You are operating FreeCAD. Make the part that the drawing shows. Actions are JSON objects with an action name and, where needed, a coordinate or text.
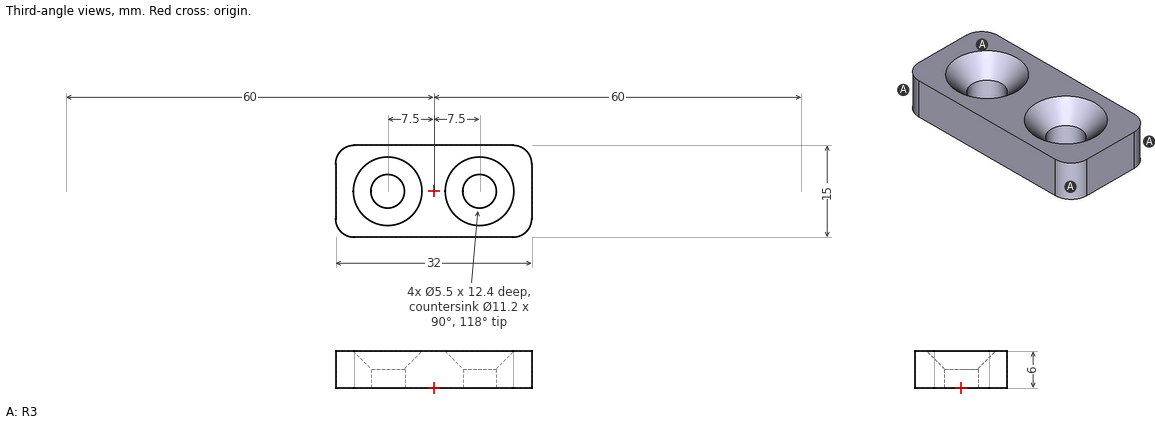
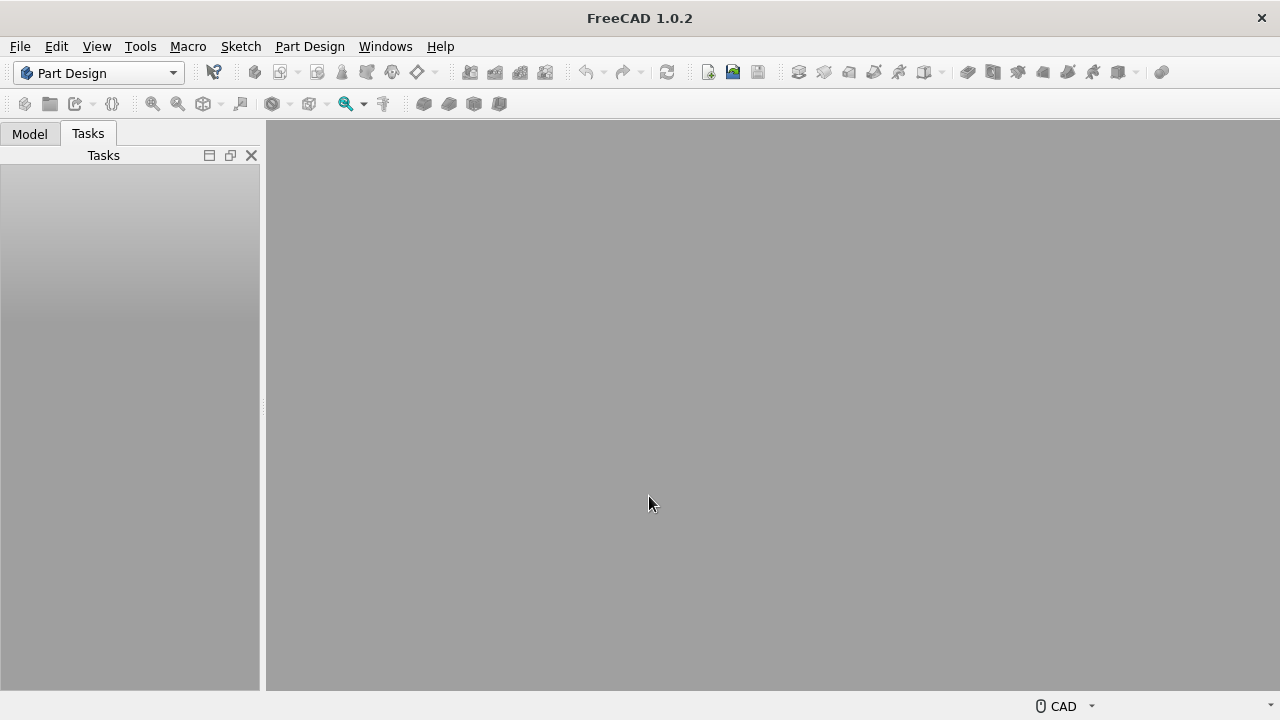
{"action": "left_click", "coordinate": [708, 72]}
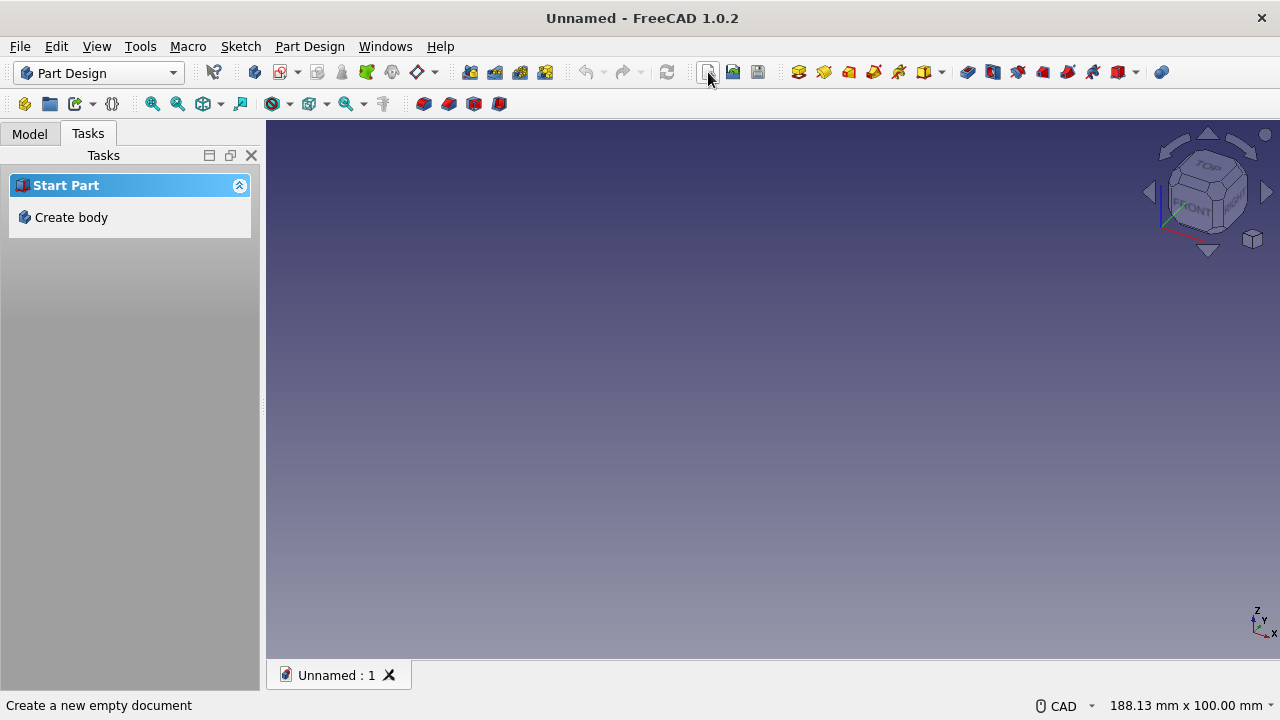
{"action": "left_click", "coordinate": [280, 72]}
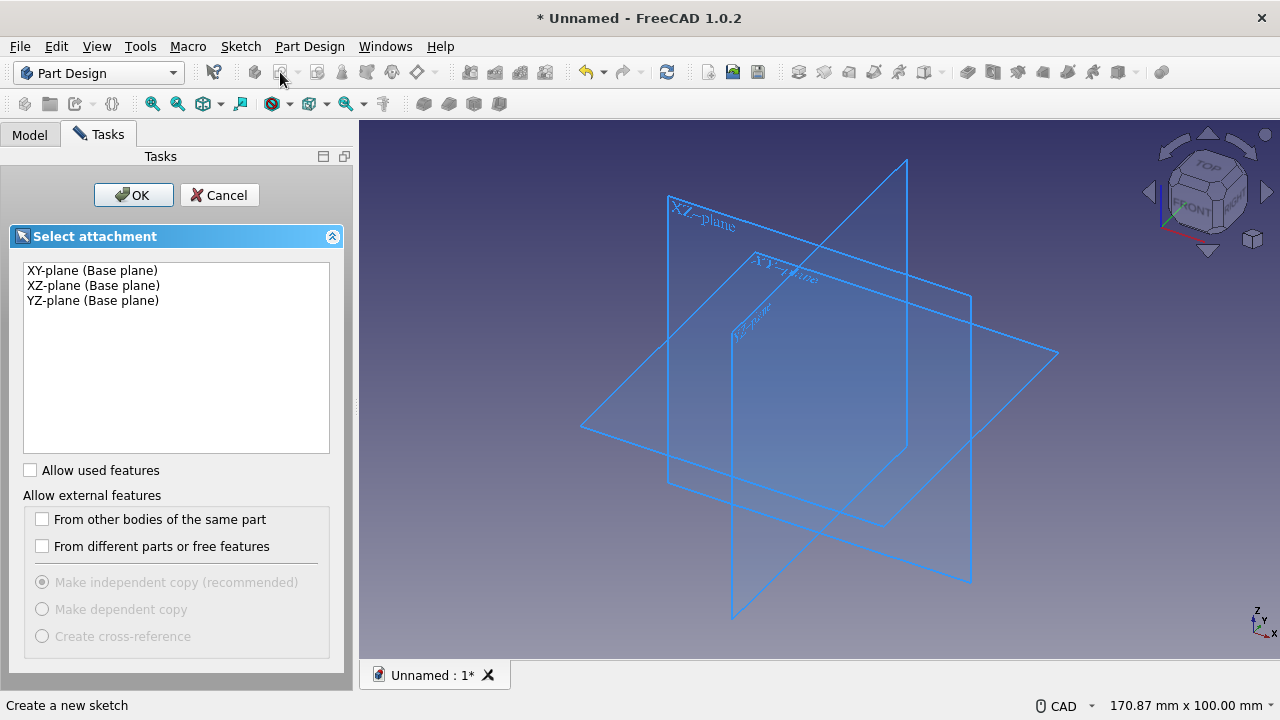
{"action": "left_click", "coordinate": [84, 270]}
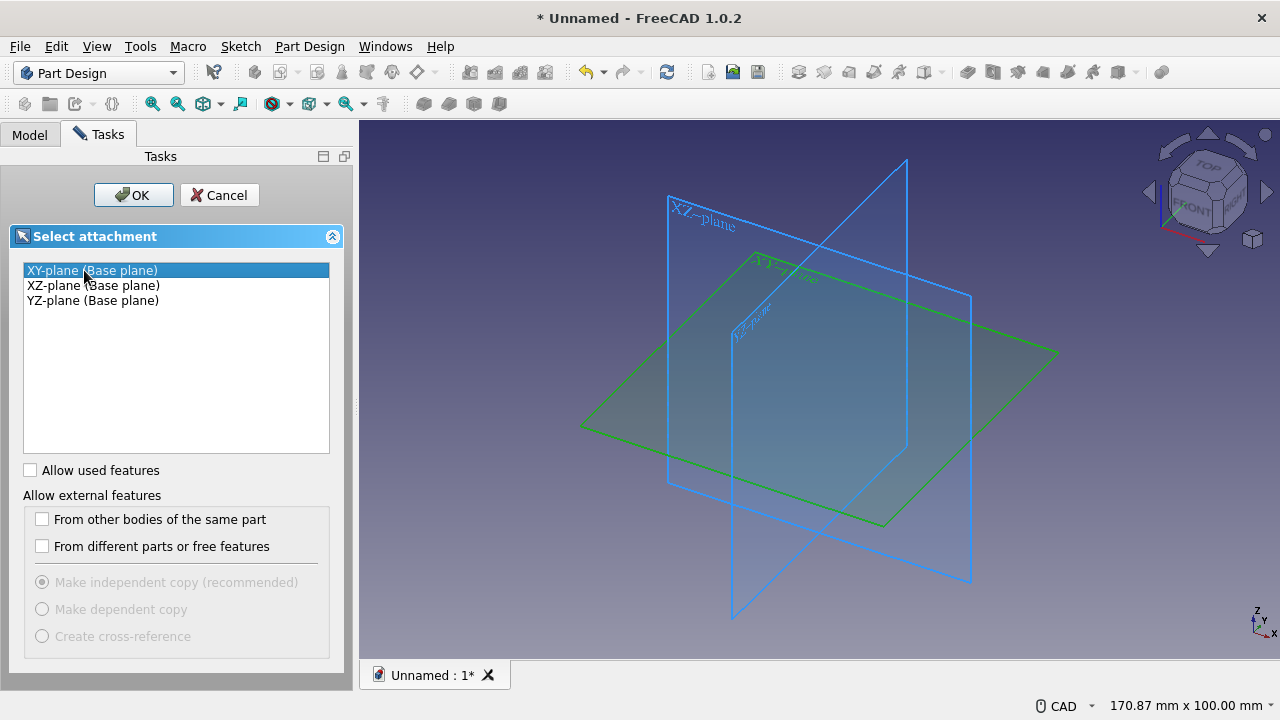
{"action": "left_click", "coordinate": [134, 195]}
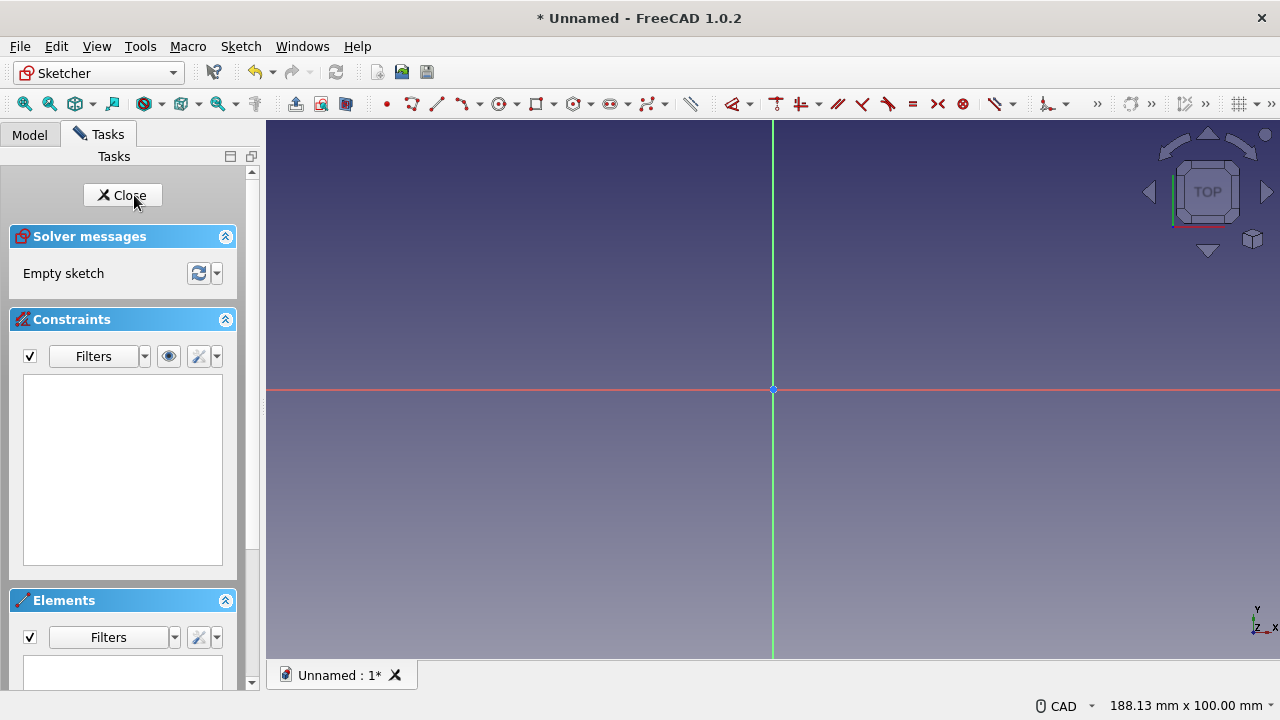
{"action": "scroll", "coordinate": [803, 390], "scroll_direction": "up", "scroll_amount": 6}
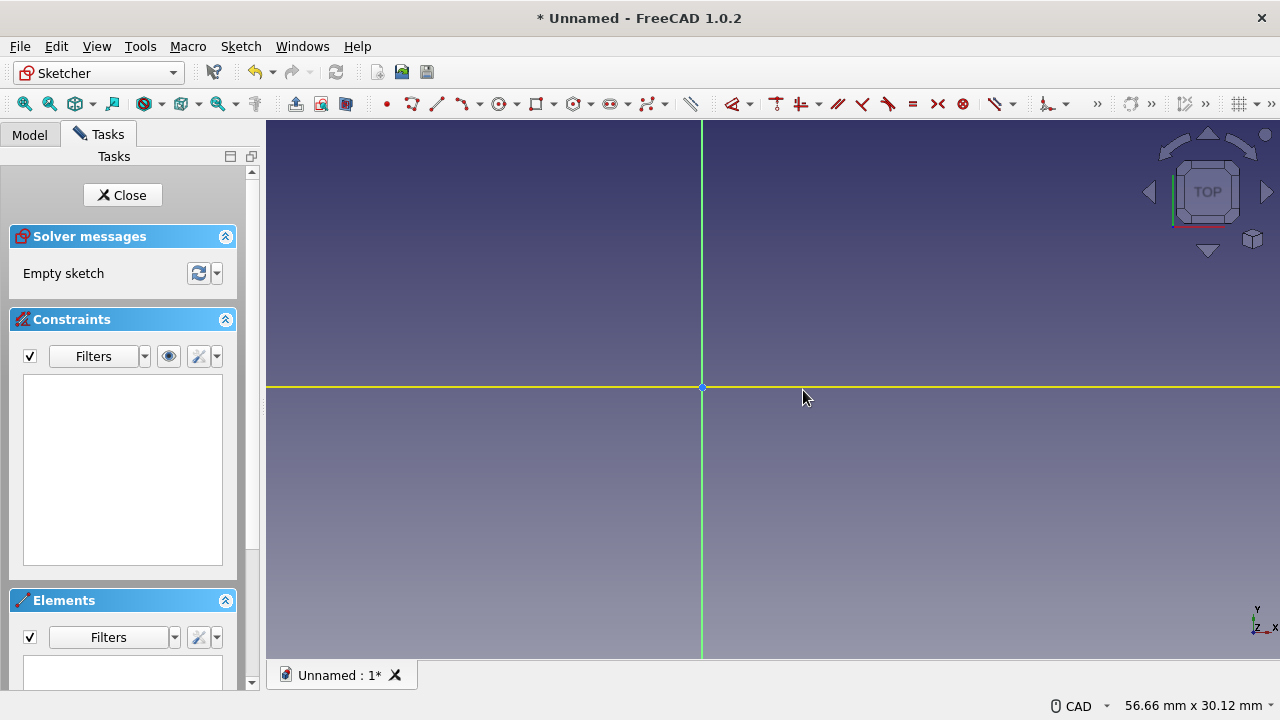
{"action": "key", "text": "g v"}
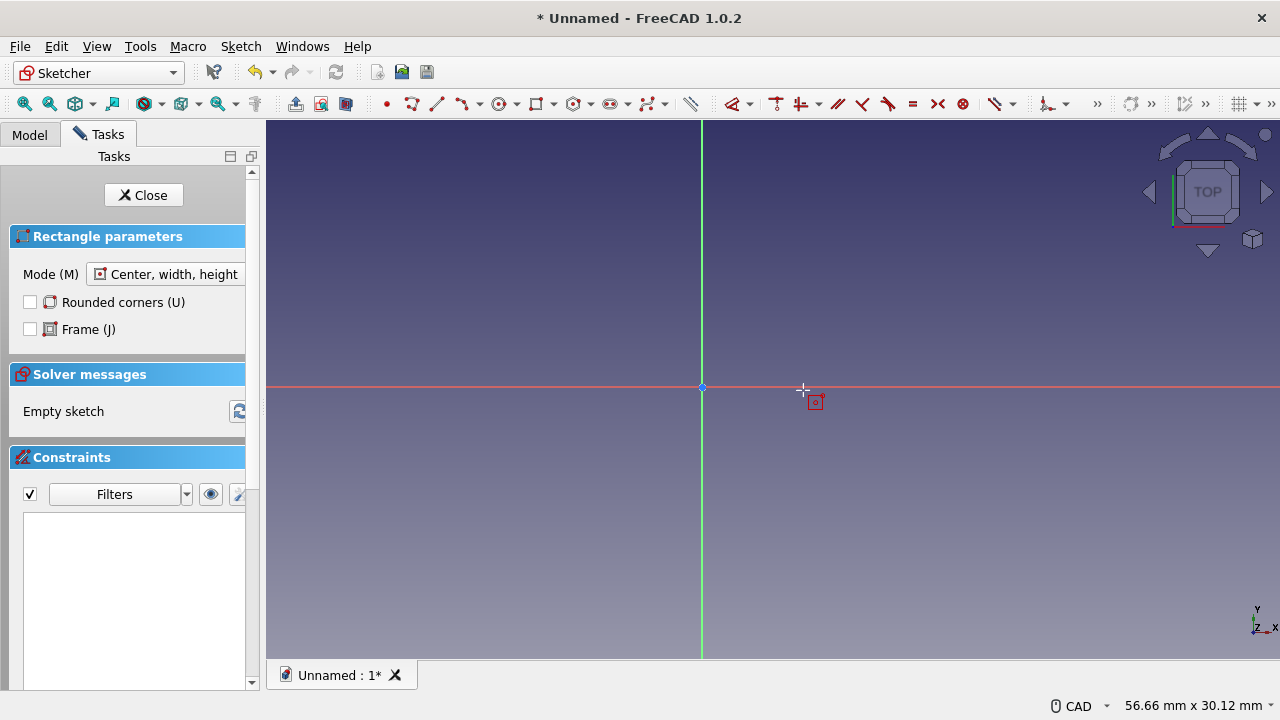
{"action": "left_click", "coordinate": [702, 387]}
{"action": "mouse_move", "coordinate": [988, 253]}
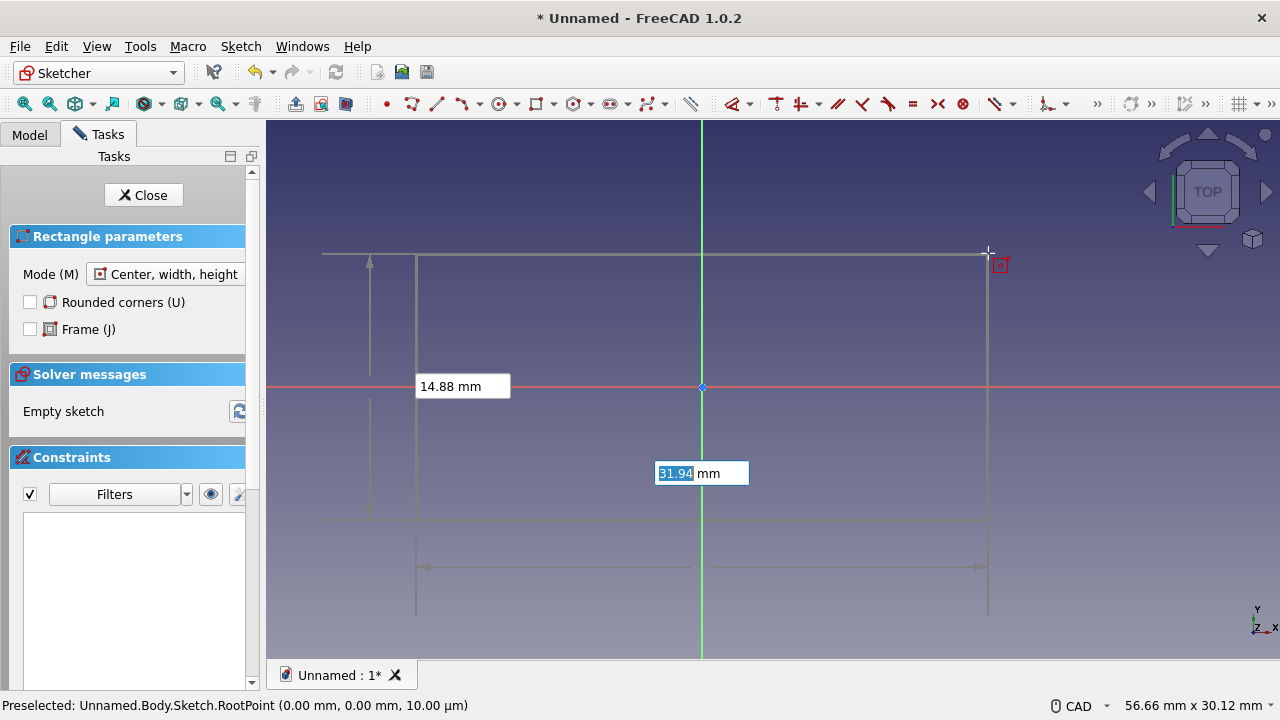
{"action": "type", "text": "32"}
{"action": "key", "text": "Tab"}
{"action": "type", "text": "15"}
{"action": "key", "text": "Return"}
{"action": "key", "text": "Escape"}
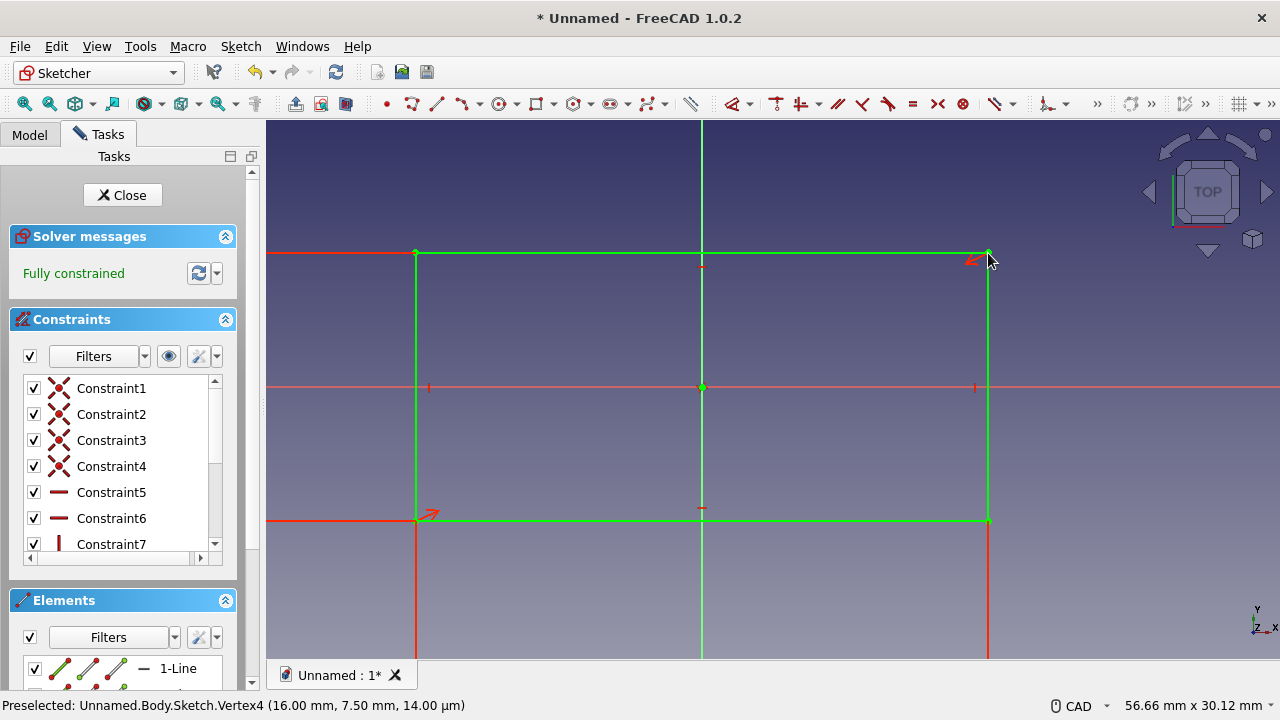
{"action": "left_click", "coordinate": [123, 195]}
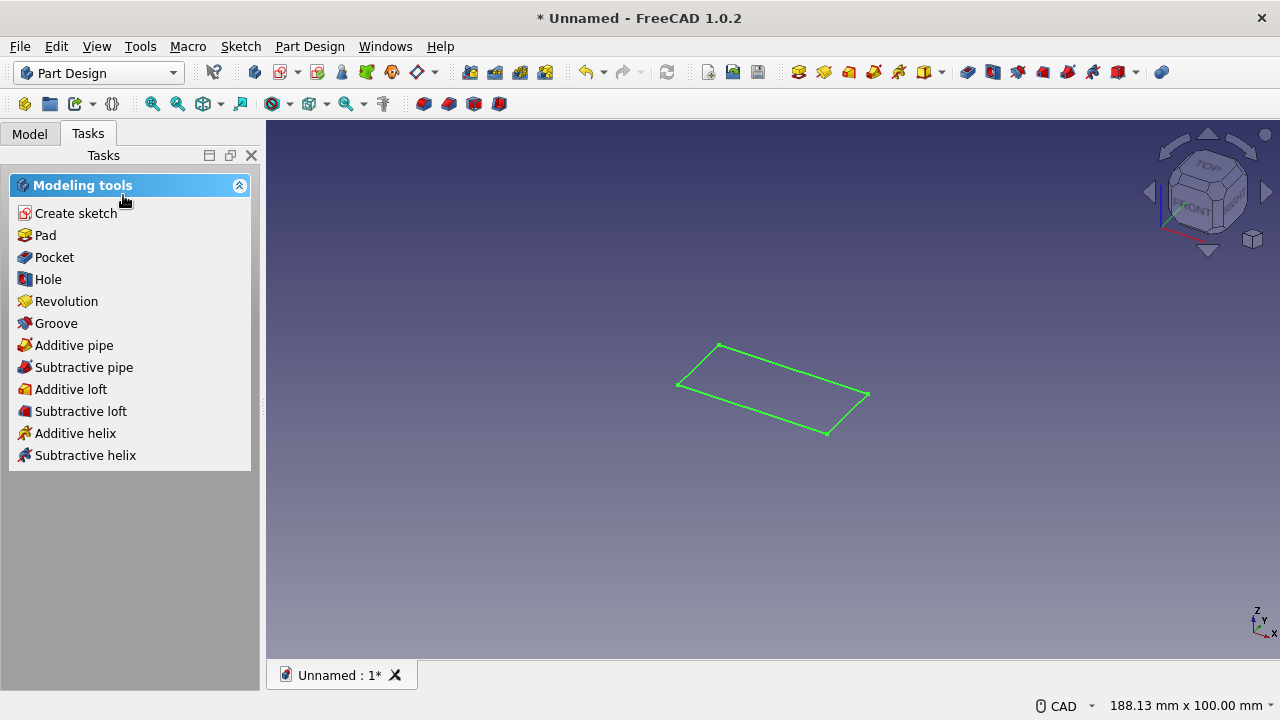
{"action": "left_click", "coordinate": [799, 72]}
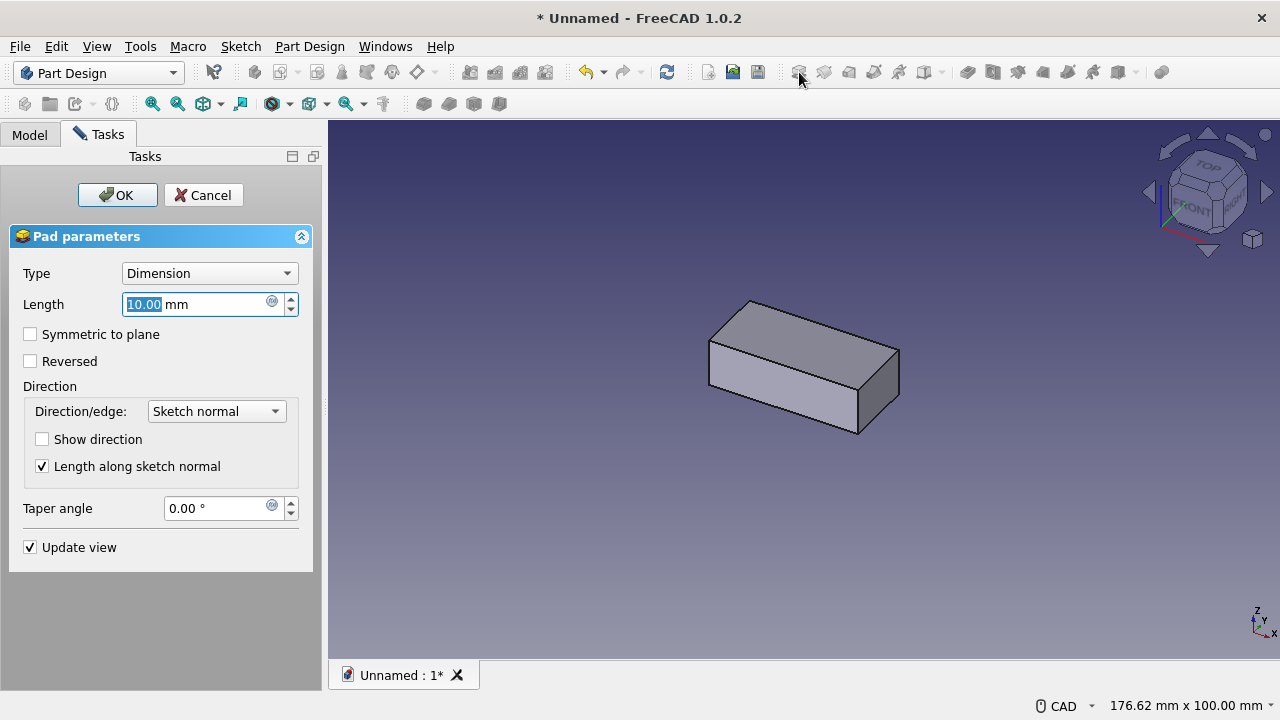
{"action": "type", "text": "6"}
{"action": "key", "text": "Tab"}